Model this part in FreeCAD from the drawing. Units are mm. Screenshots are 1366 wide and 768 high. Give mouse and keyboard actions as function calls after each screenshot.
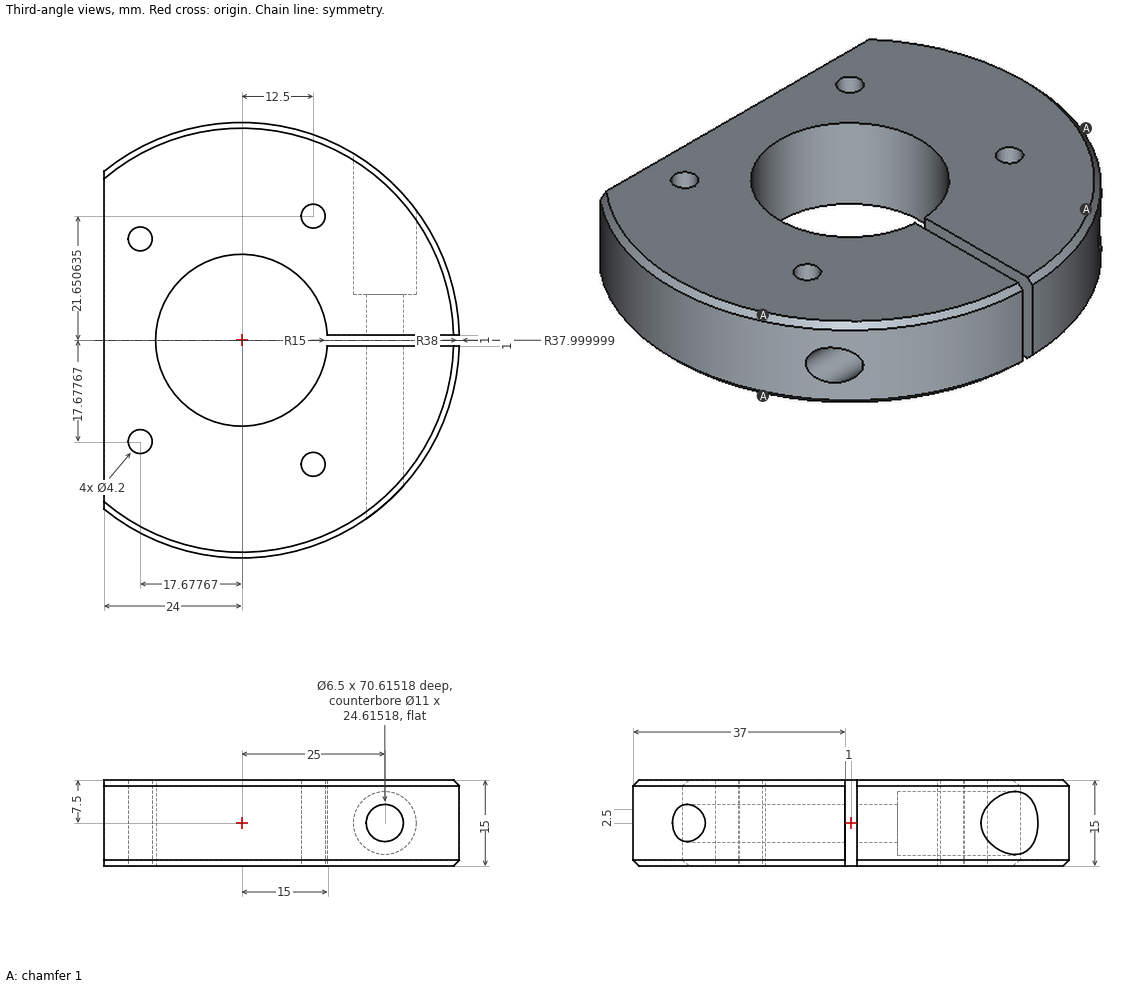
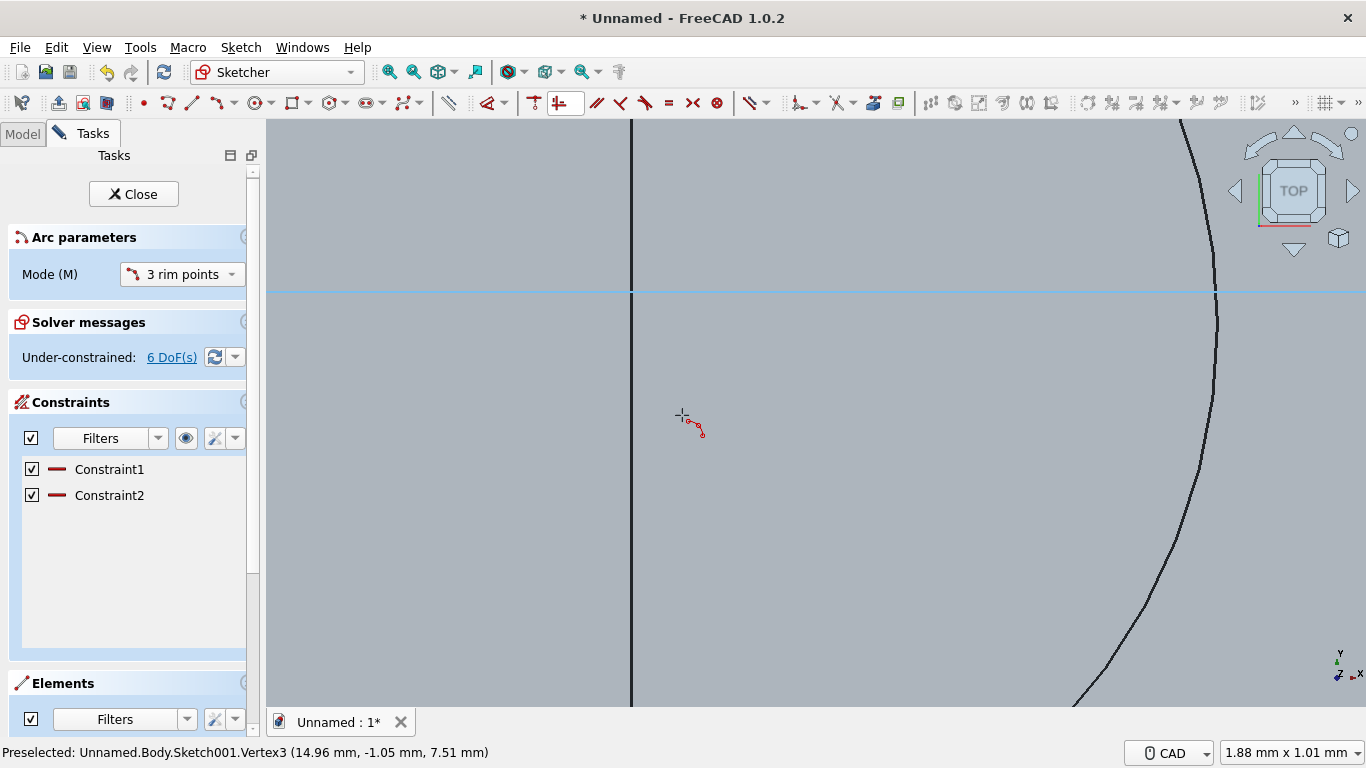
click(656, 409)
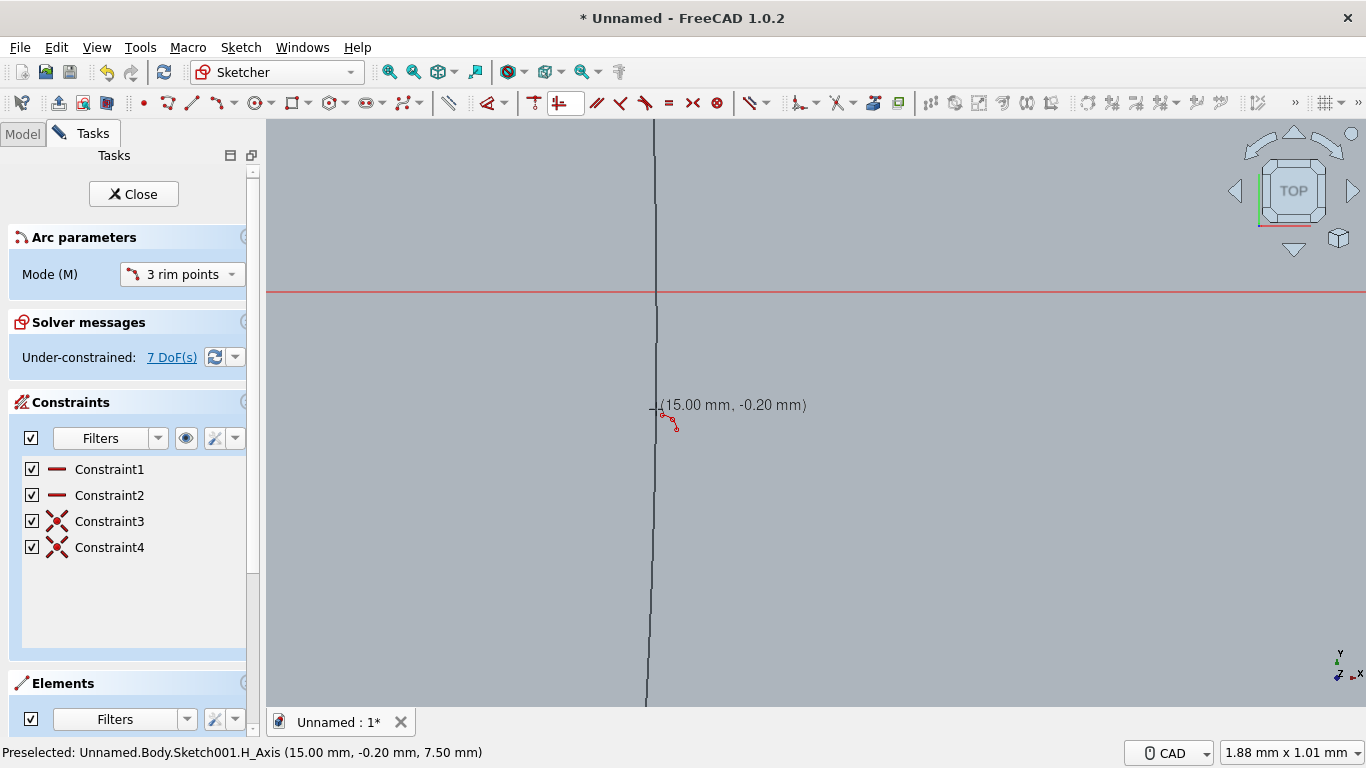
scroll(670, 417, down, 17)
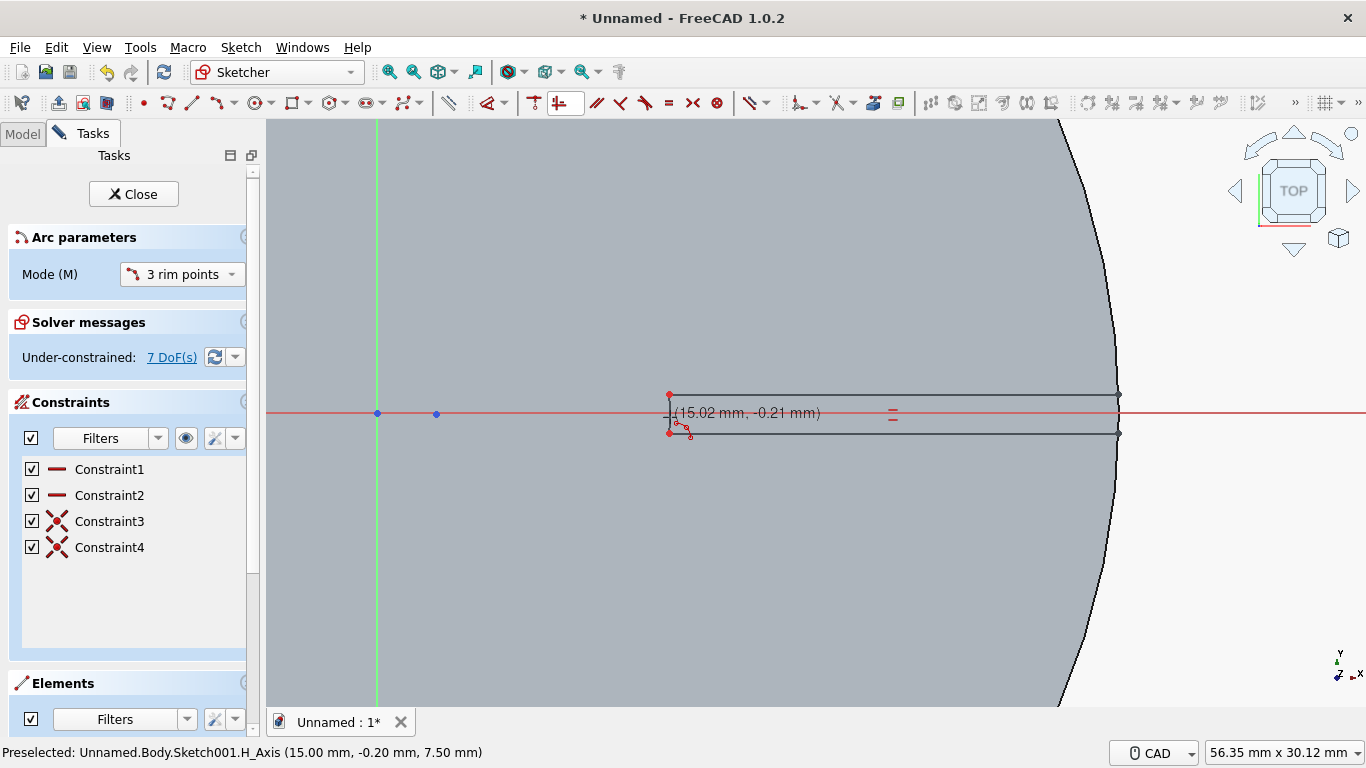
click(1119, 434)
click(1119, 395)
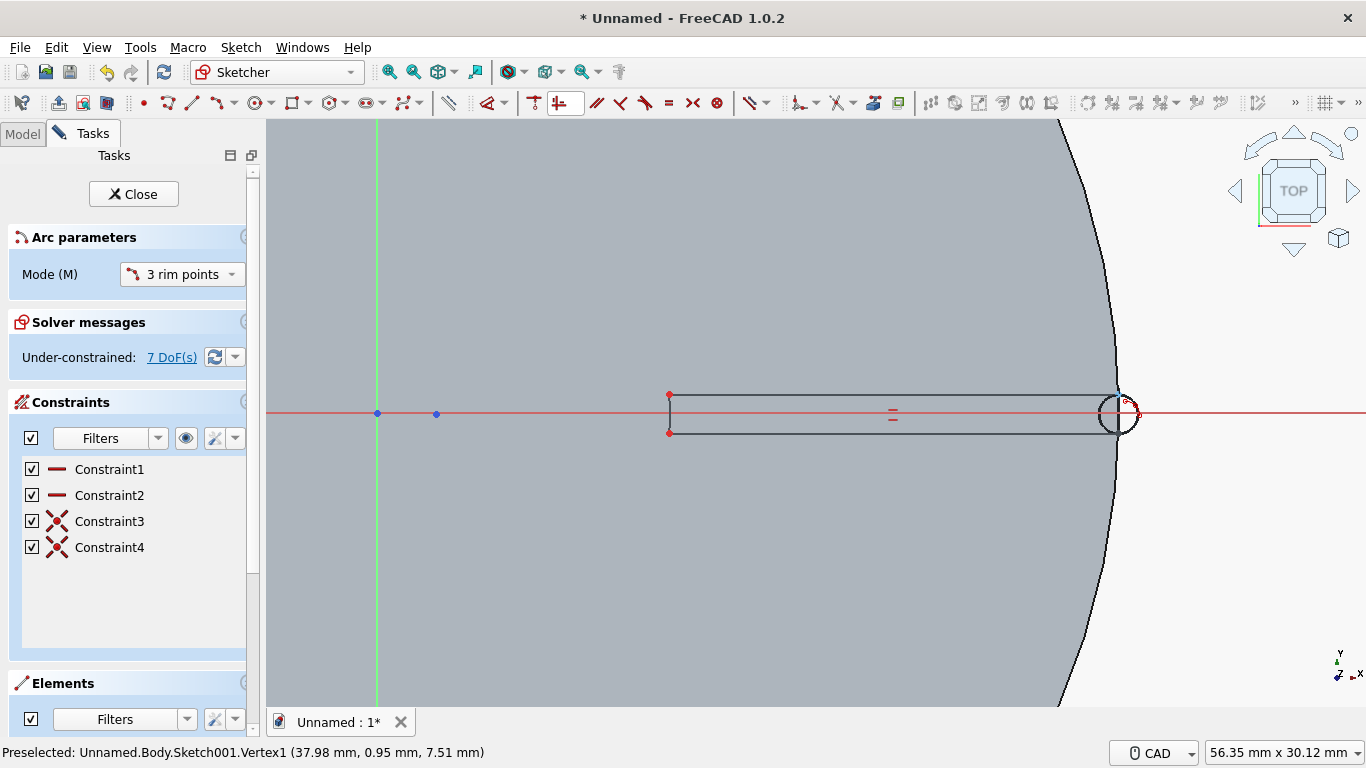
scroll(1119, 417, up, 21)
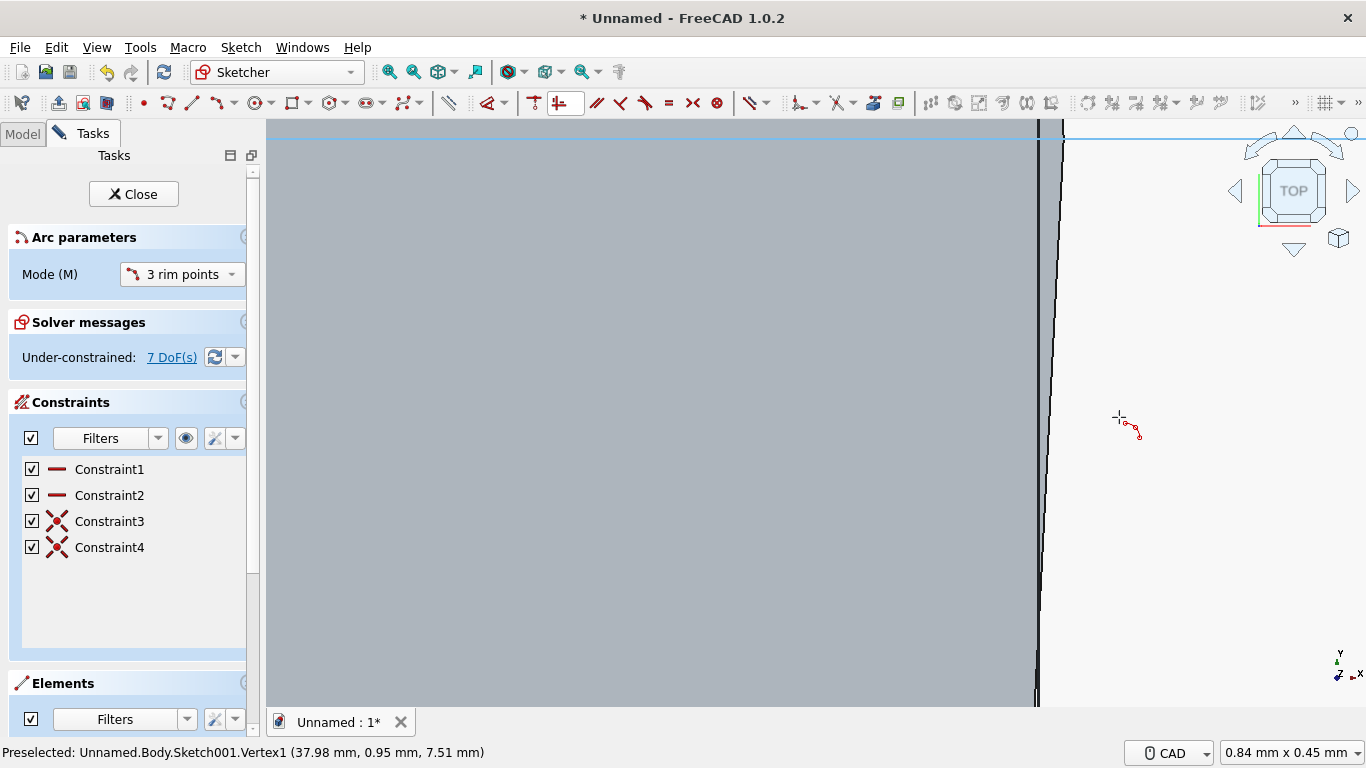
click(1063, 399)
key(Escape)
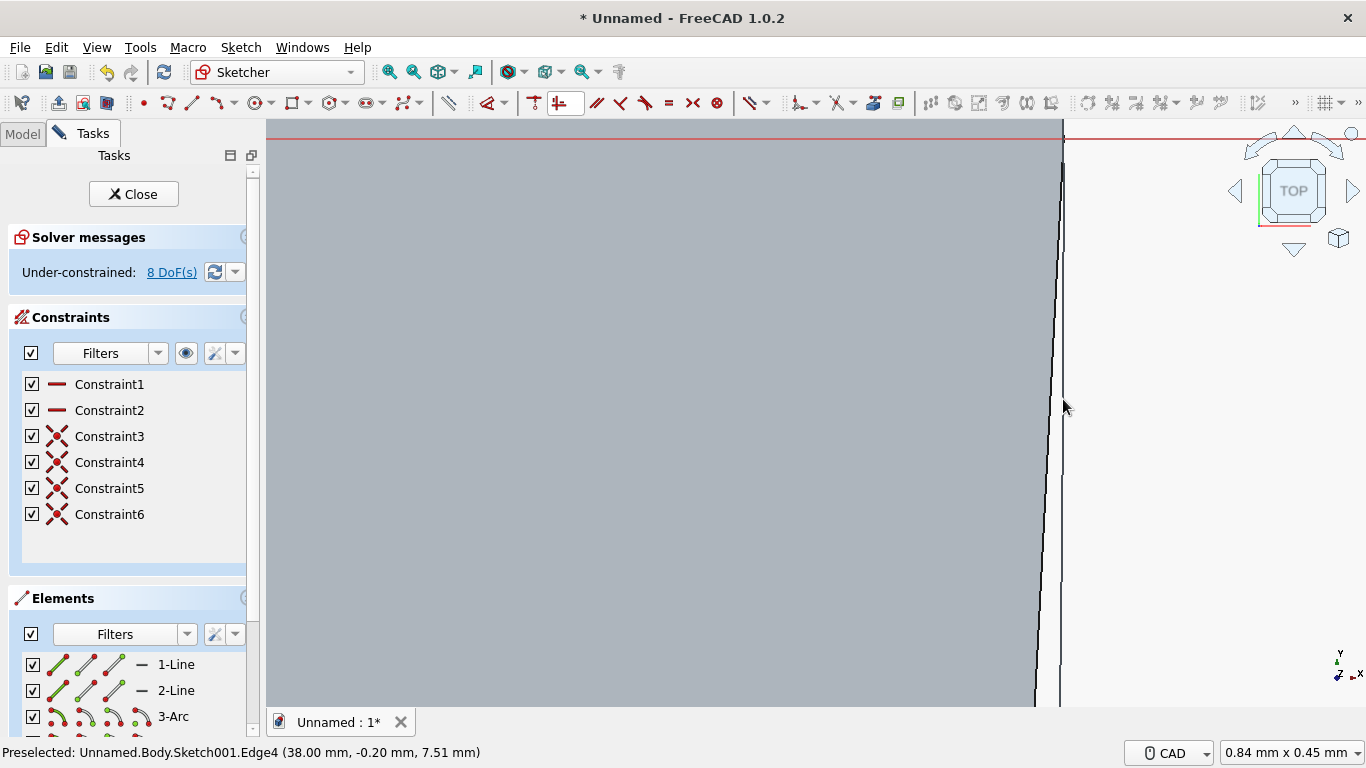
scroll(748, 413, down, 15)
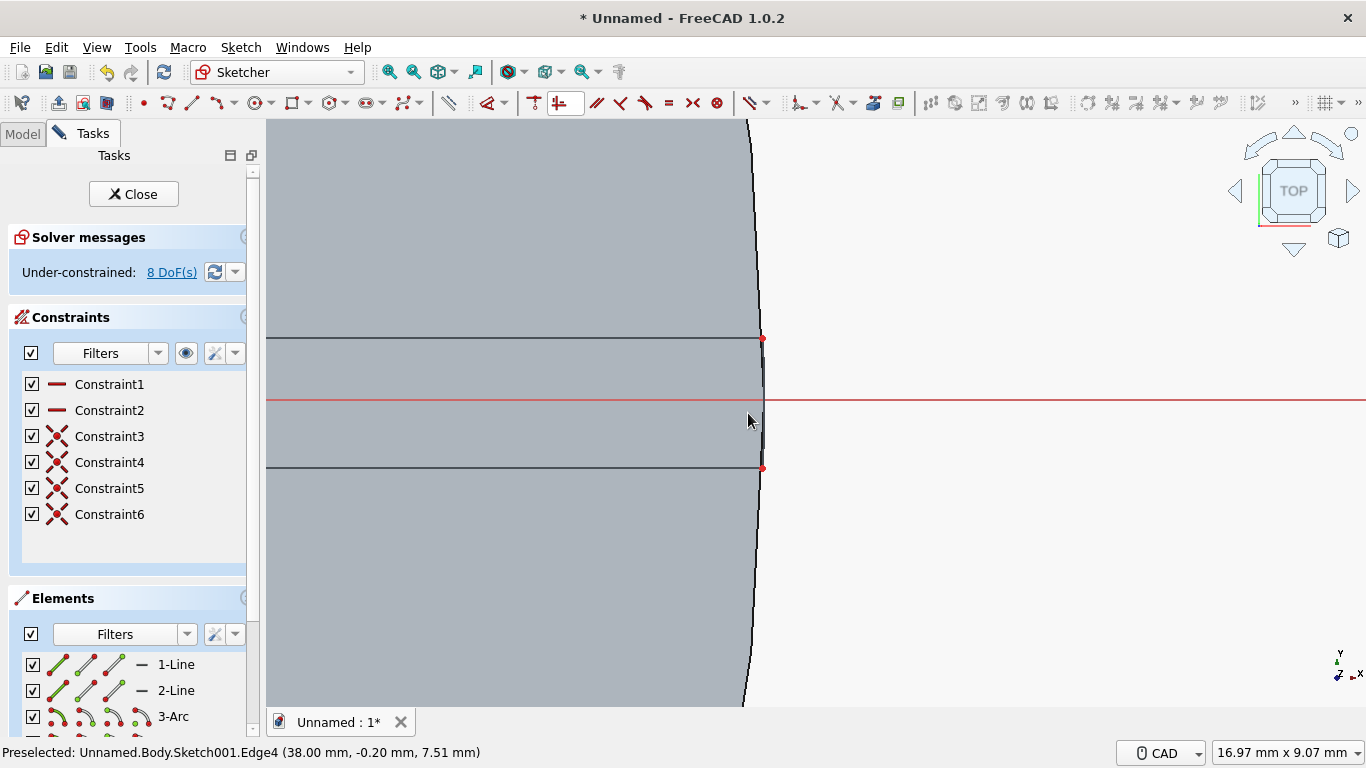
scroll(1145, 417, down, 7)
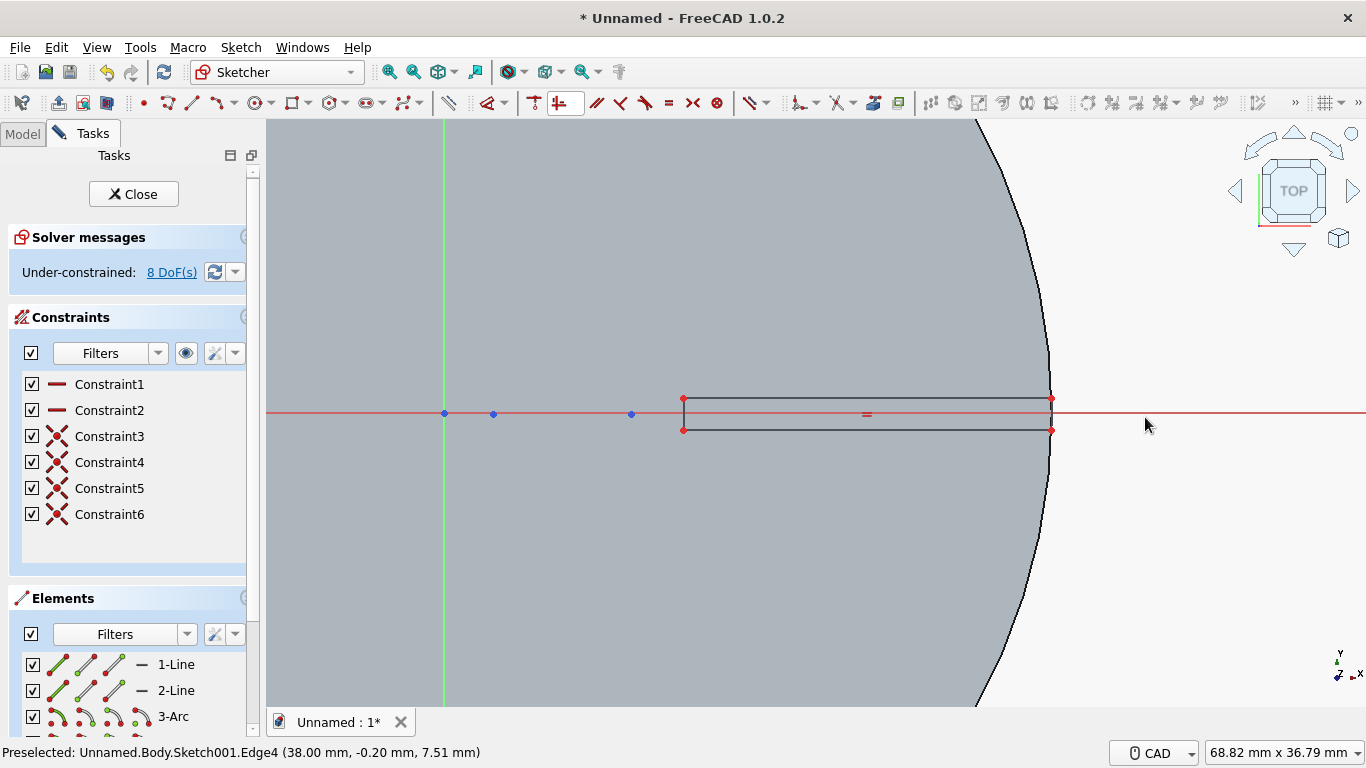
scroll(684, 420, up, 4)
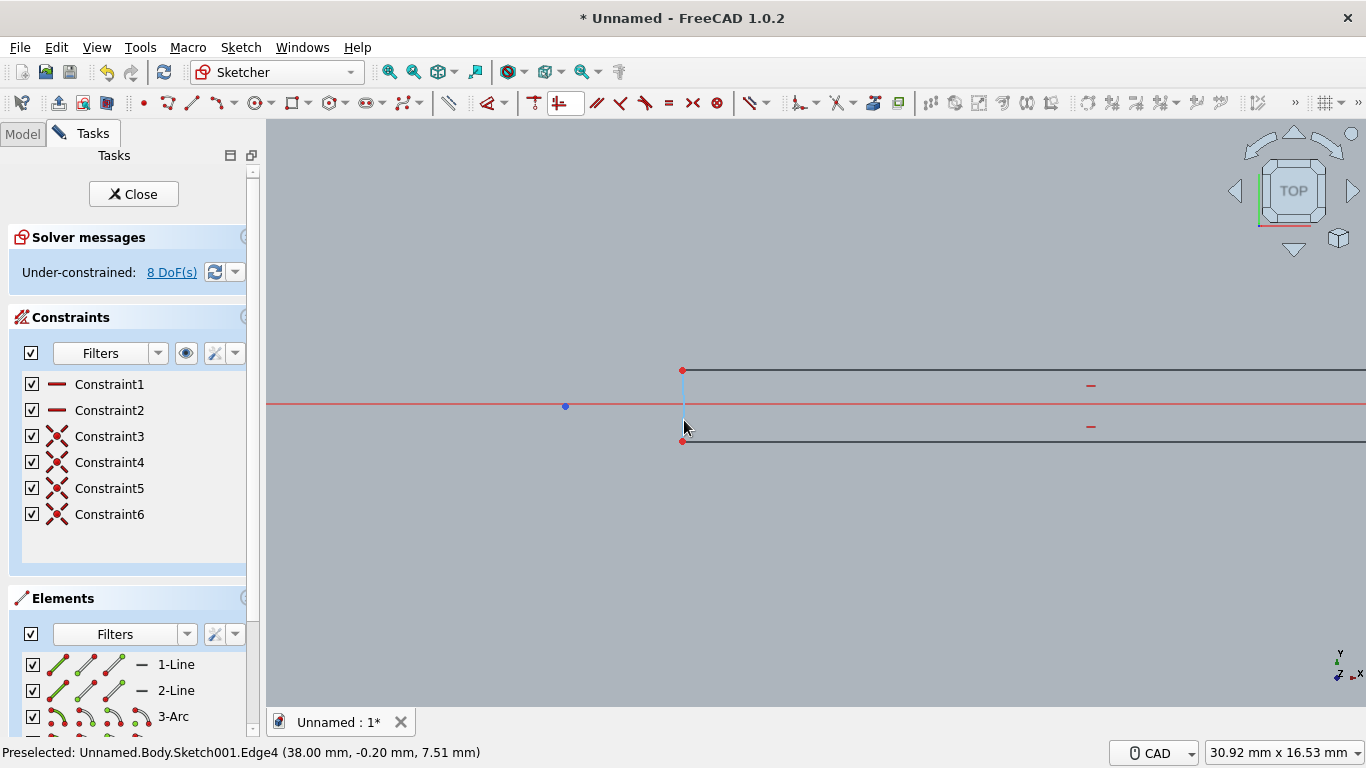
click(683, 420)